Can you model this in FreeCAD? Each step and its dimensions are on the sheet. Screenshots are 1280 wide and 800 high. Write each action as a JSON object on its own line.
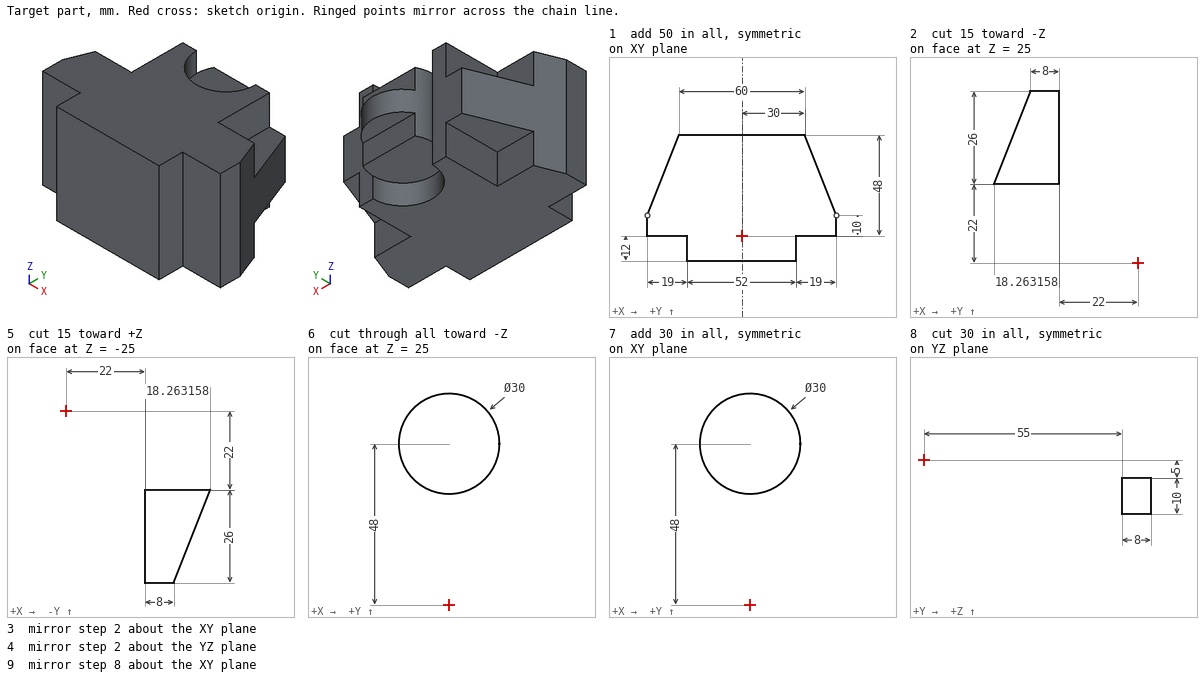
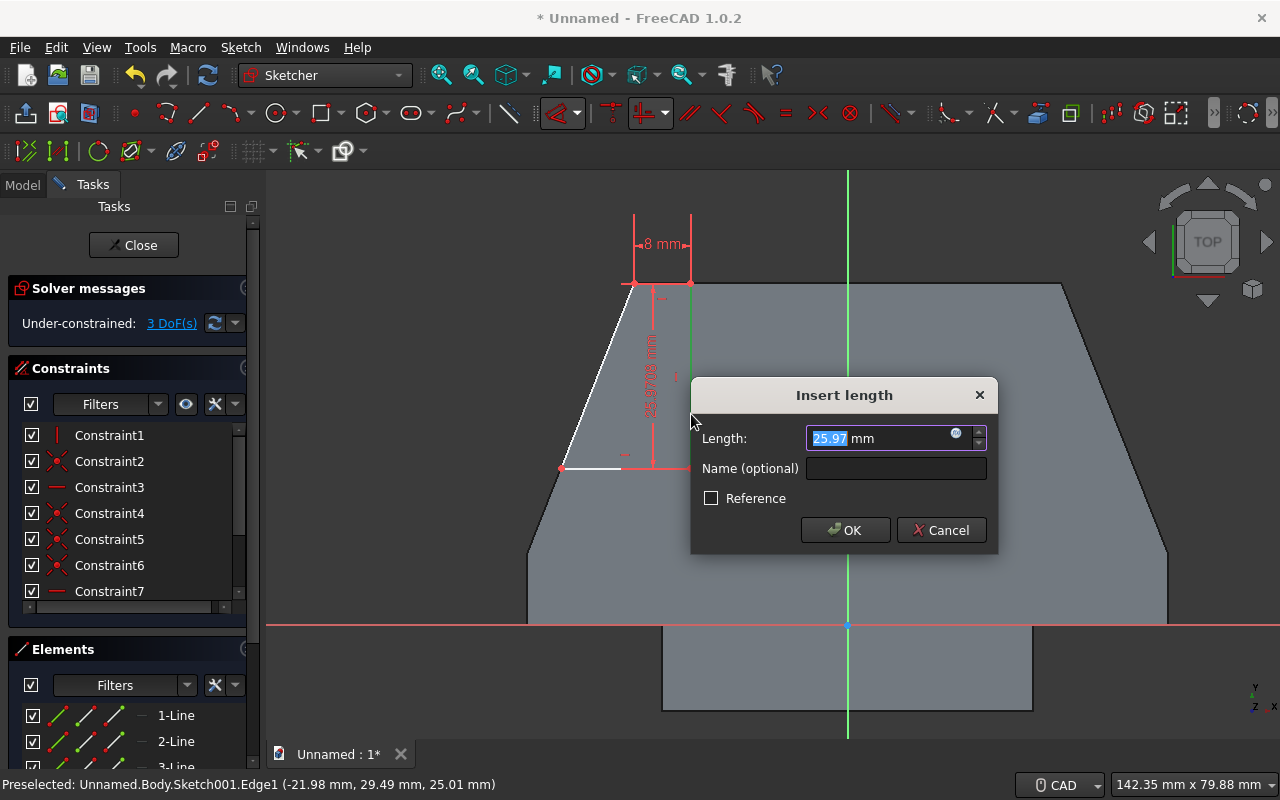
{"action": "type", "text": "26"}
{"action": "key", "text": "Return"}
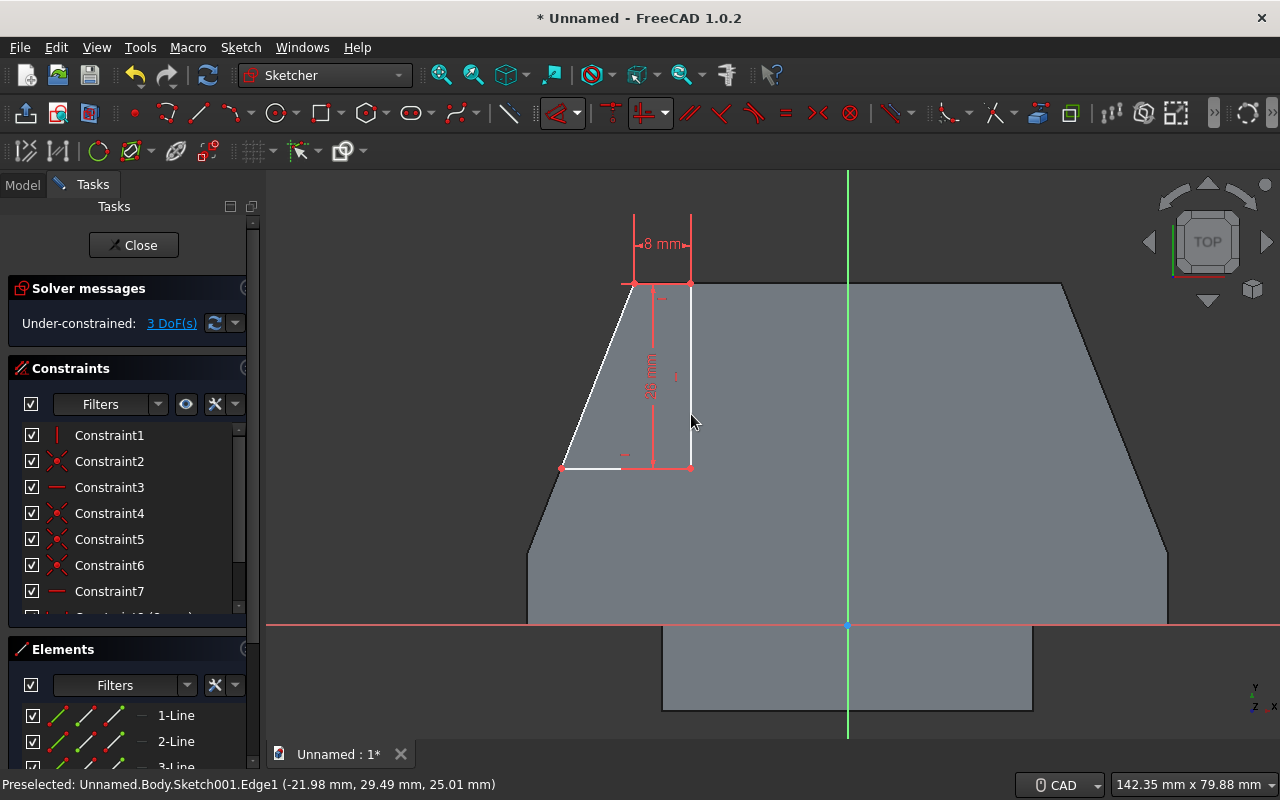
{"action": "left_click", "coordinate": [691, 469]}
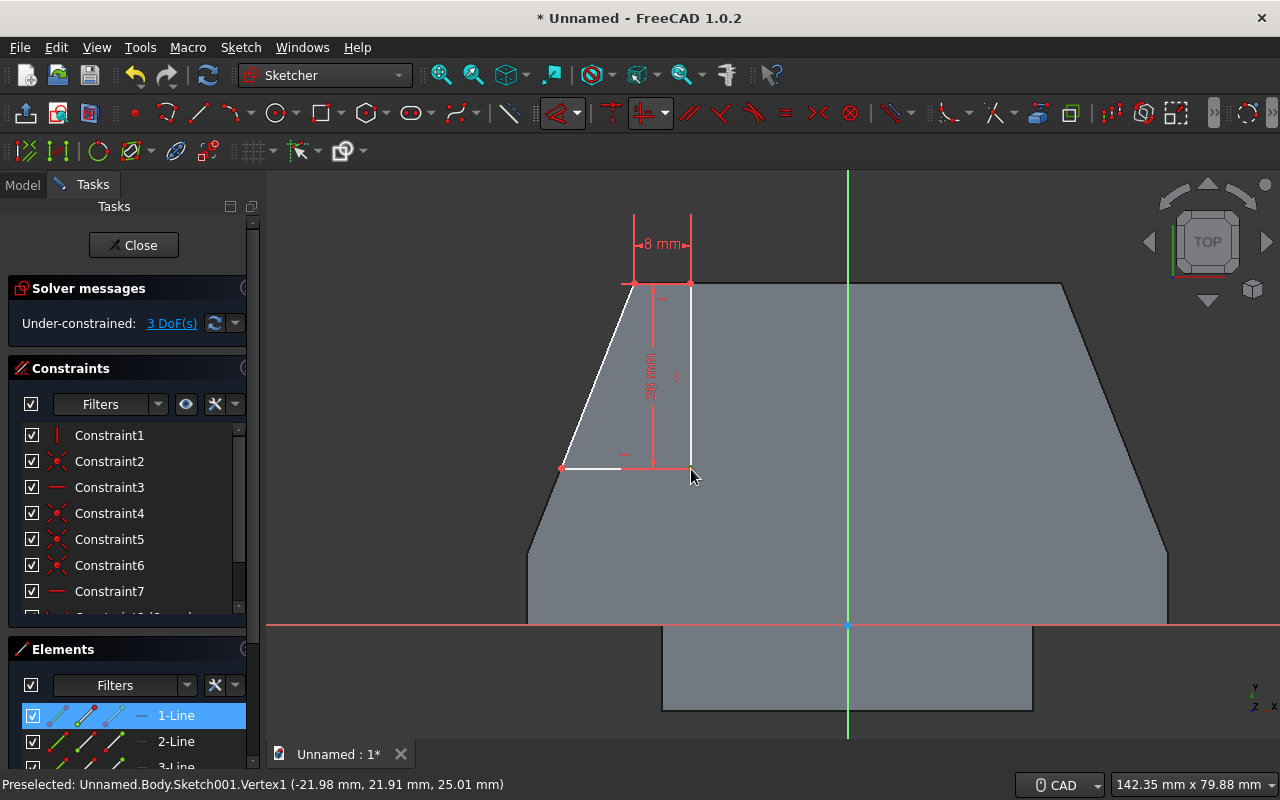
{"action": "key", "text": "l"}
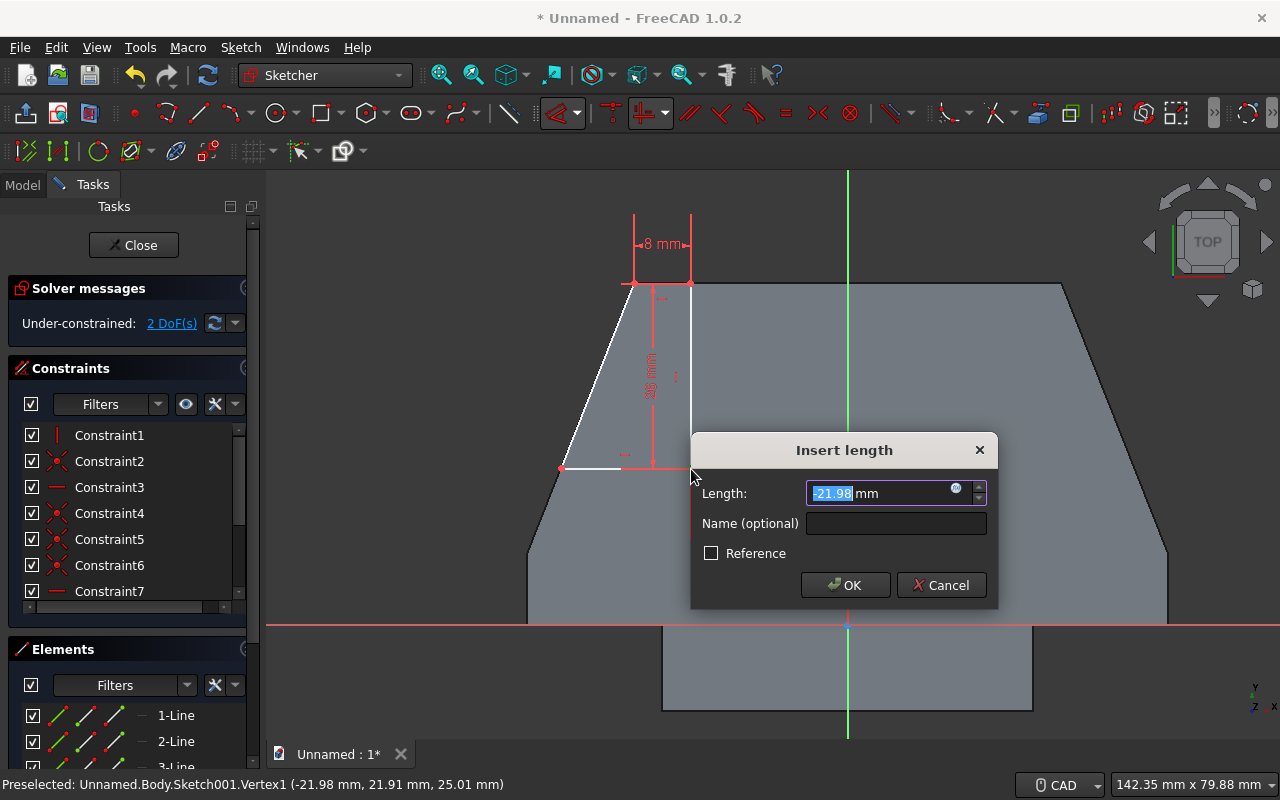
{"action": "type", "text": "-22"}
{"action": "key", "text": "Return"}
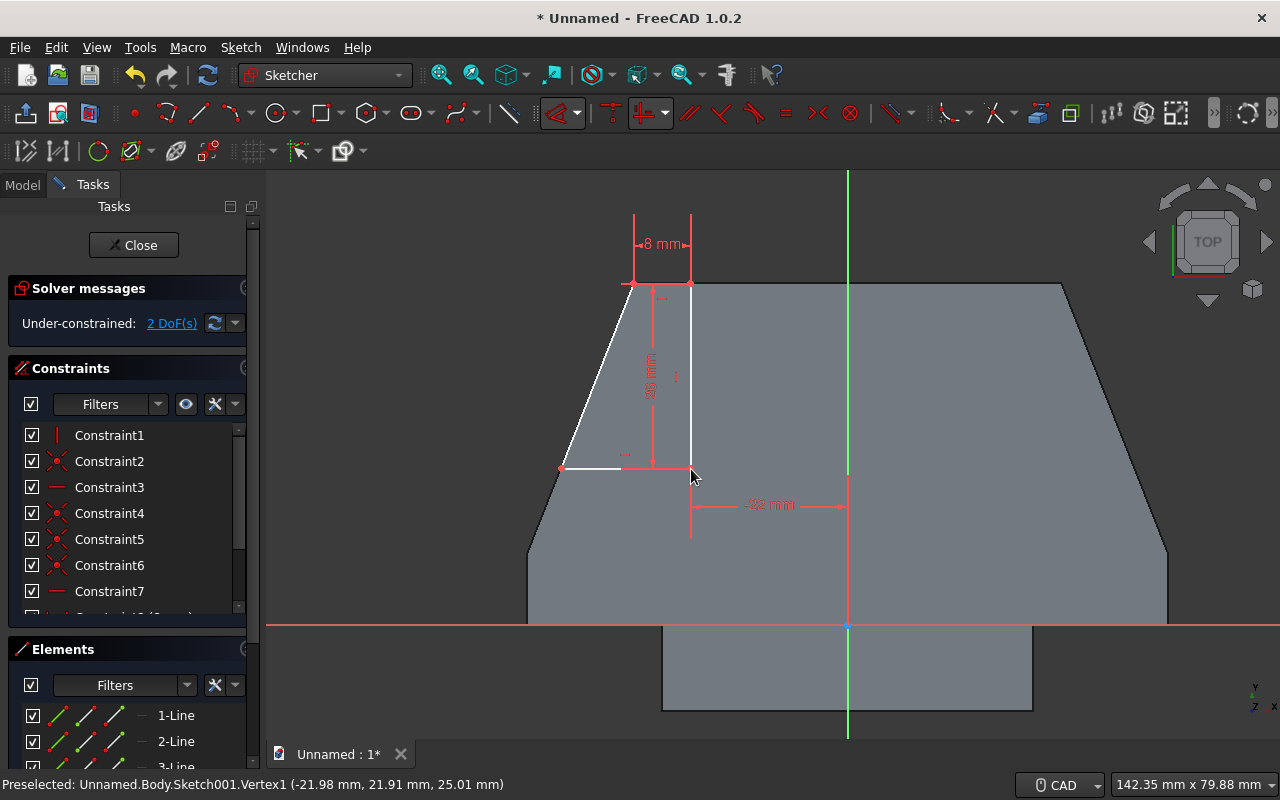
{"action": "left_click", "coordinate": [691, 469]}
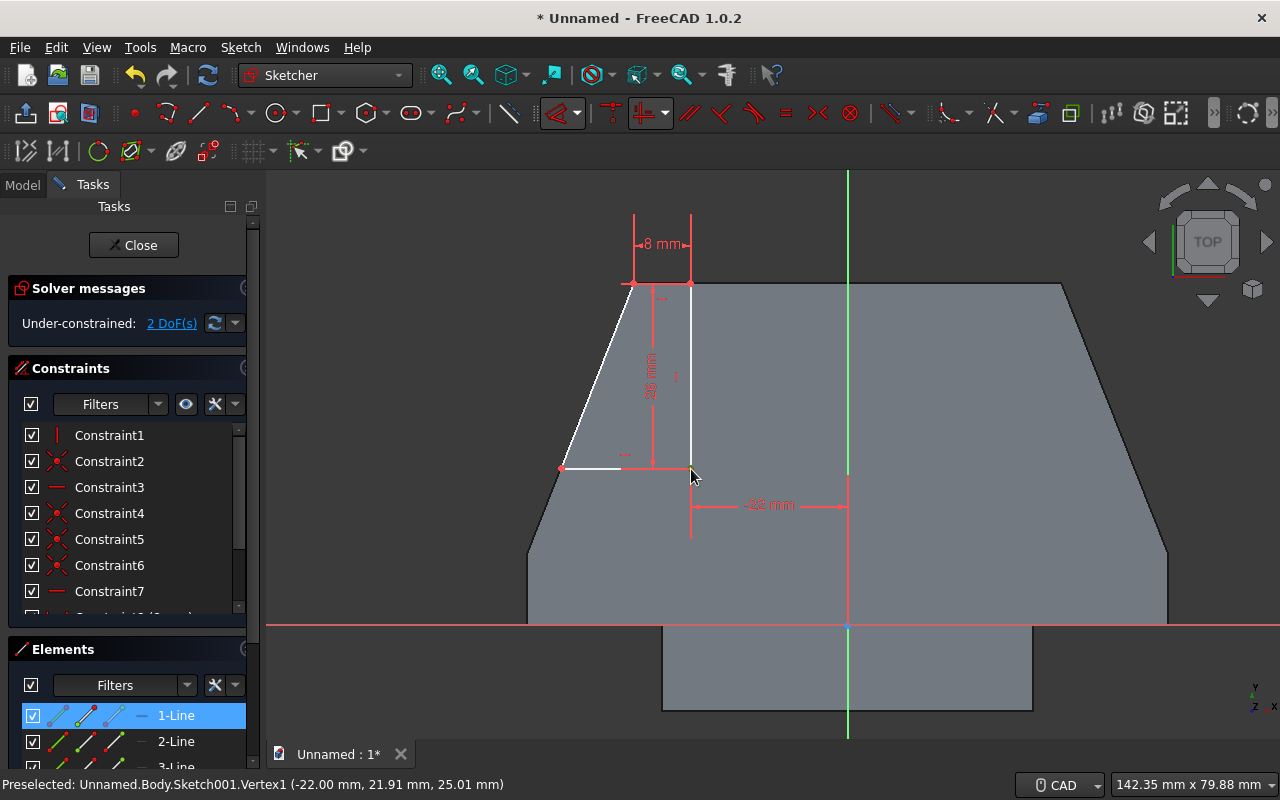
{"action": "left_click", "coordinate": [580, 114]}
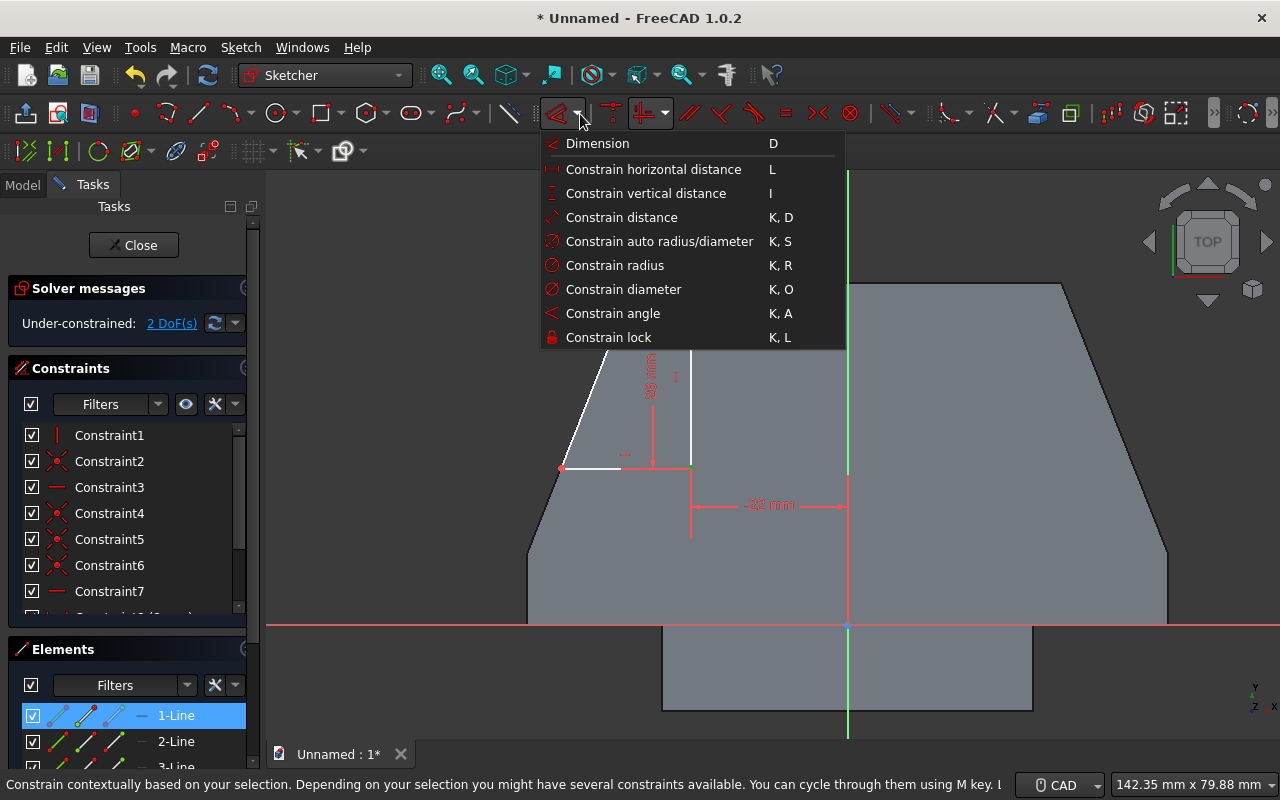
{"action": "left_click", "coordinate": [693, 193]}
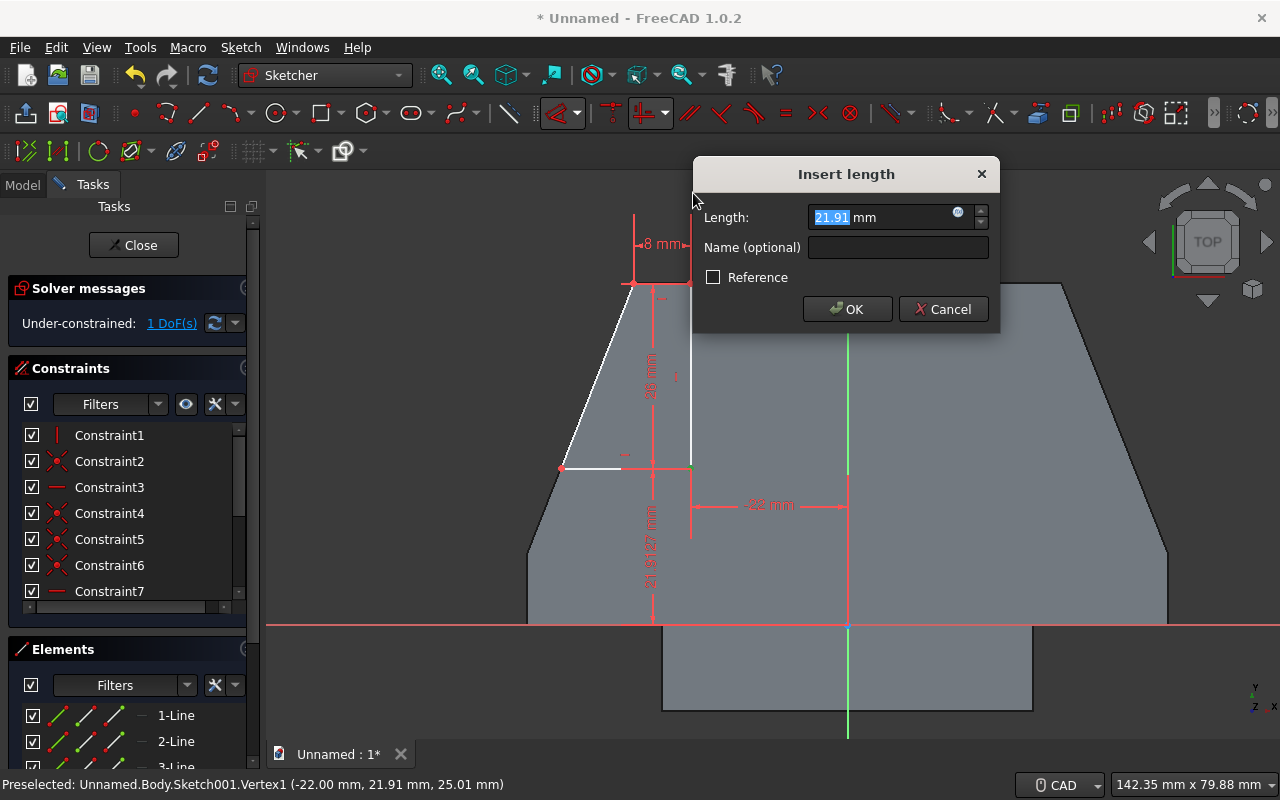
{"action": "type", "text": "22"}
{"action": "key", "text": "Return"}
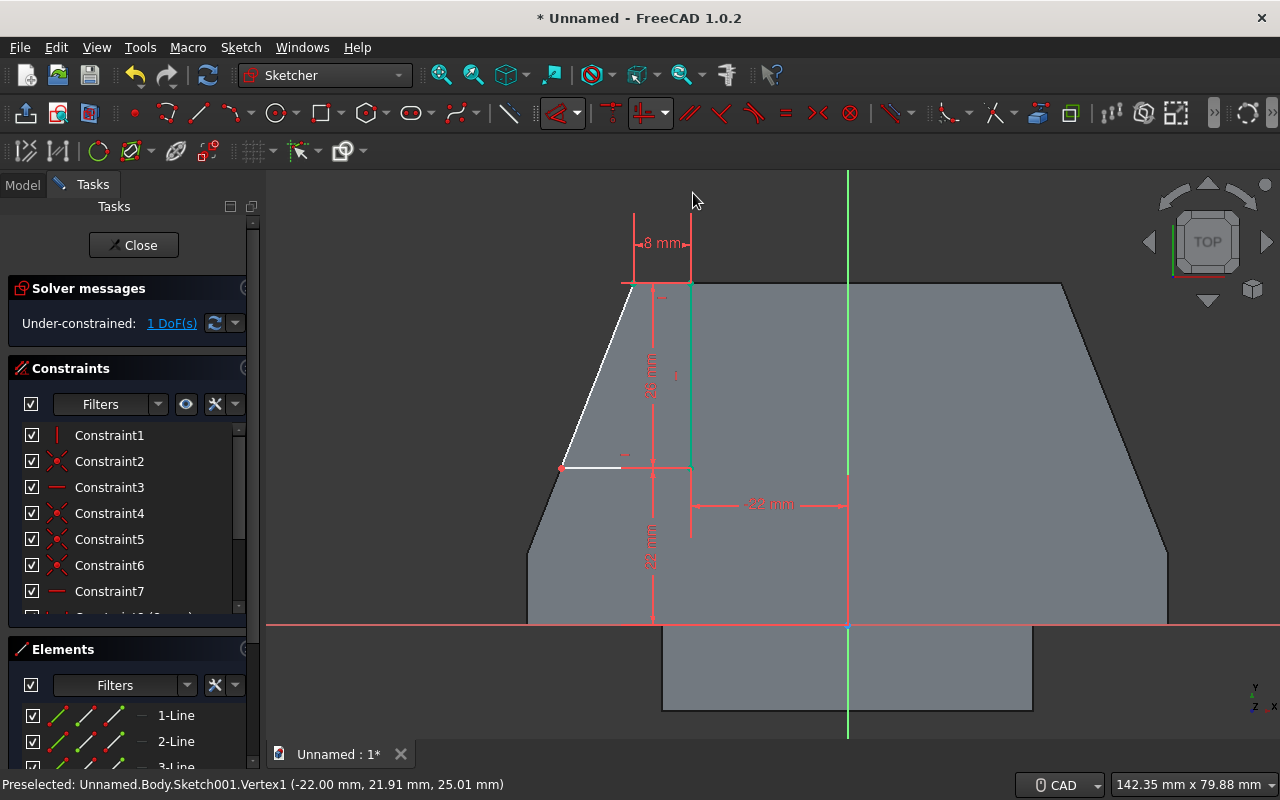
{"action": "left_click", "coordinate": [600, 468]}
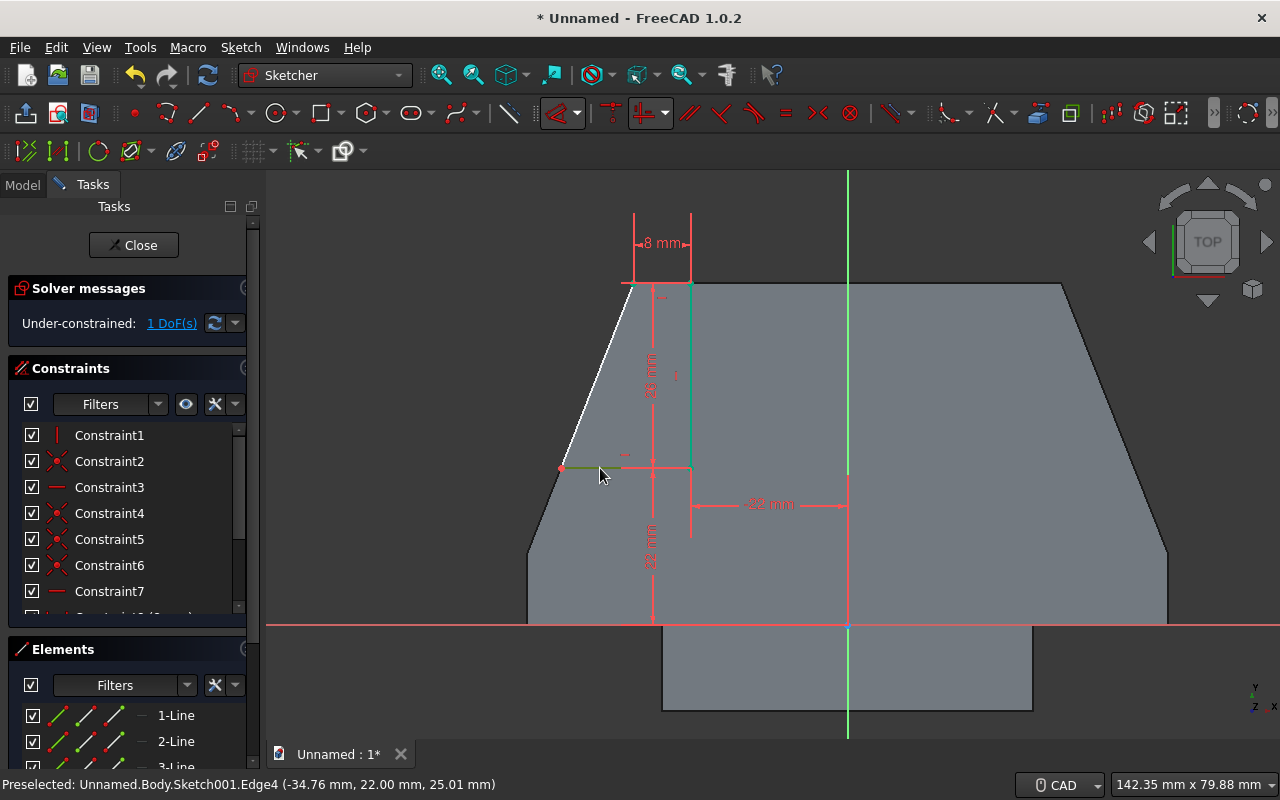
{"action": "key", "text": "l"}